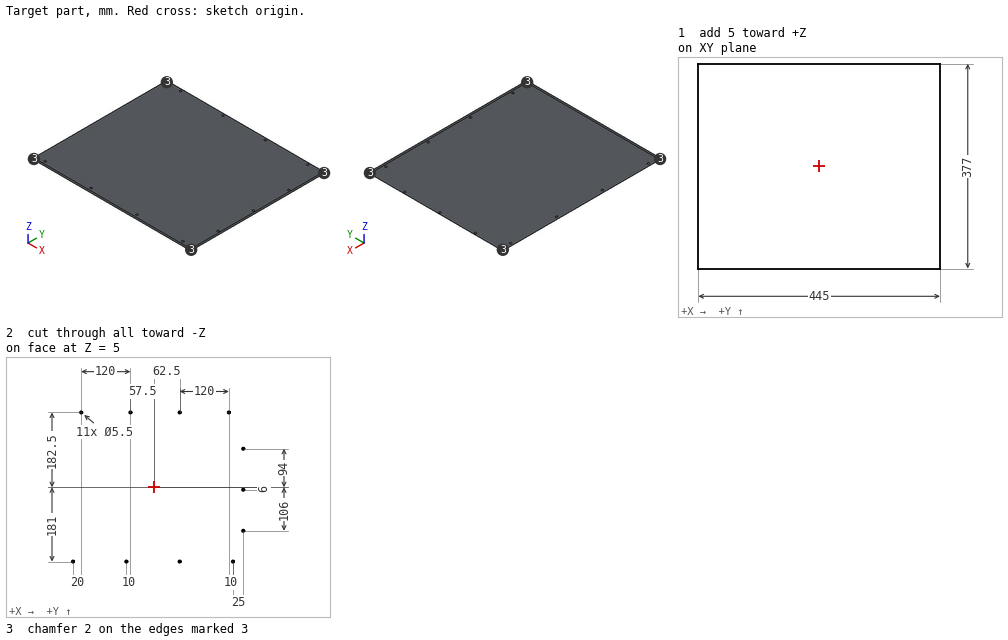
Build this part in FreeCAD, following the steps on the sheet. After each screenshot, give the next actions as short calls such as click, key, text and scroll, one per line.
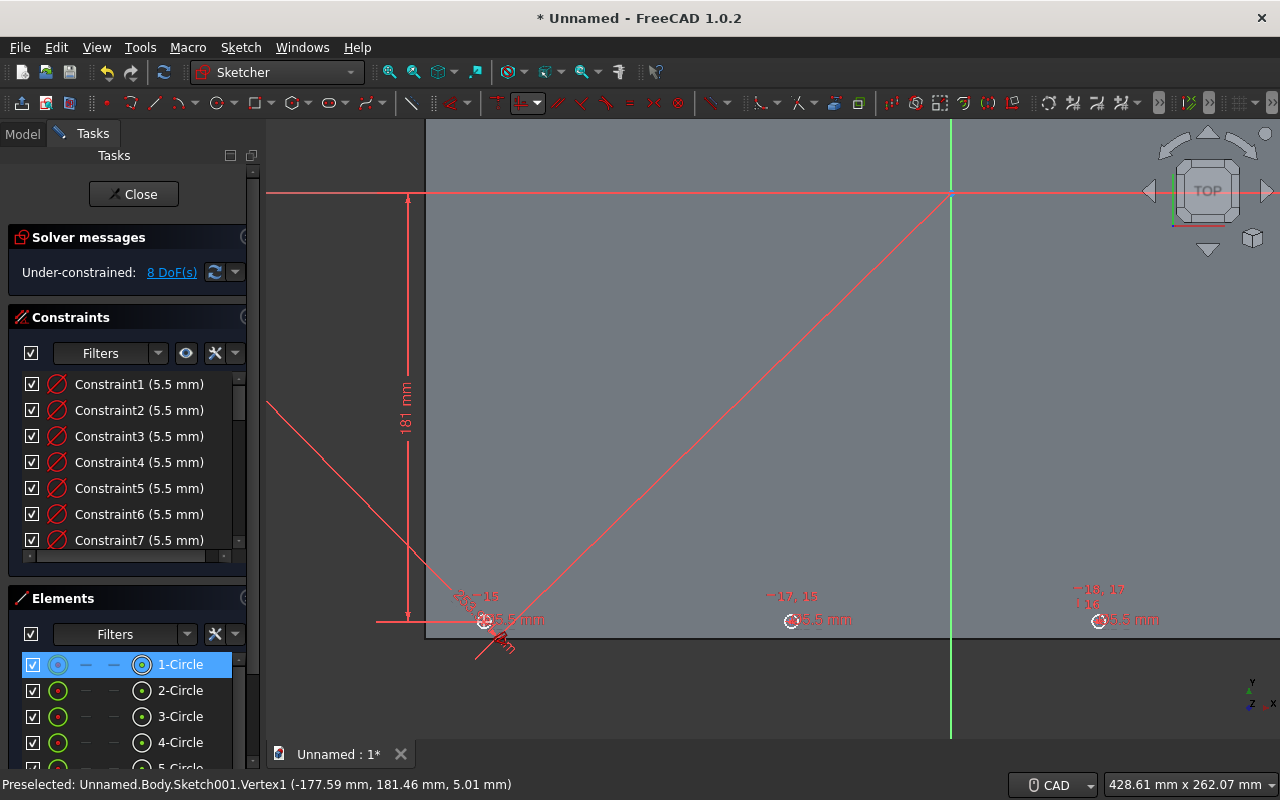
click(484, 622)
click(508, 656)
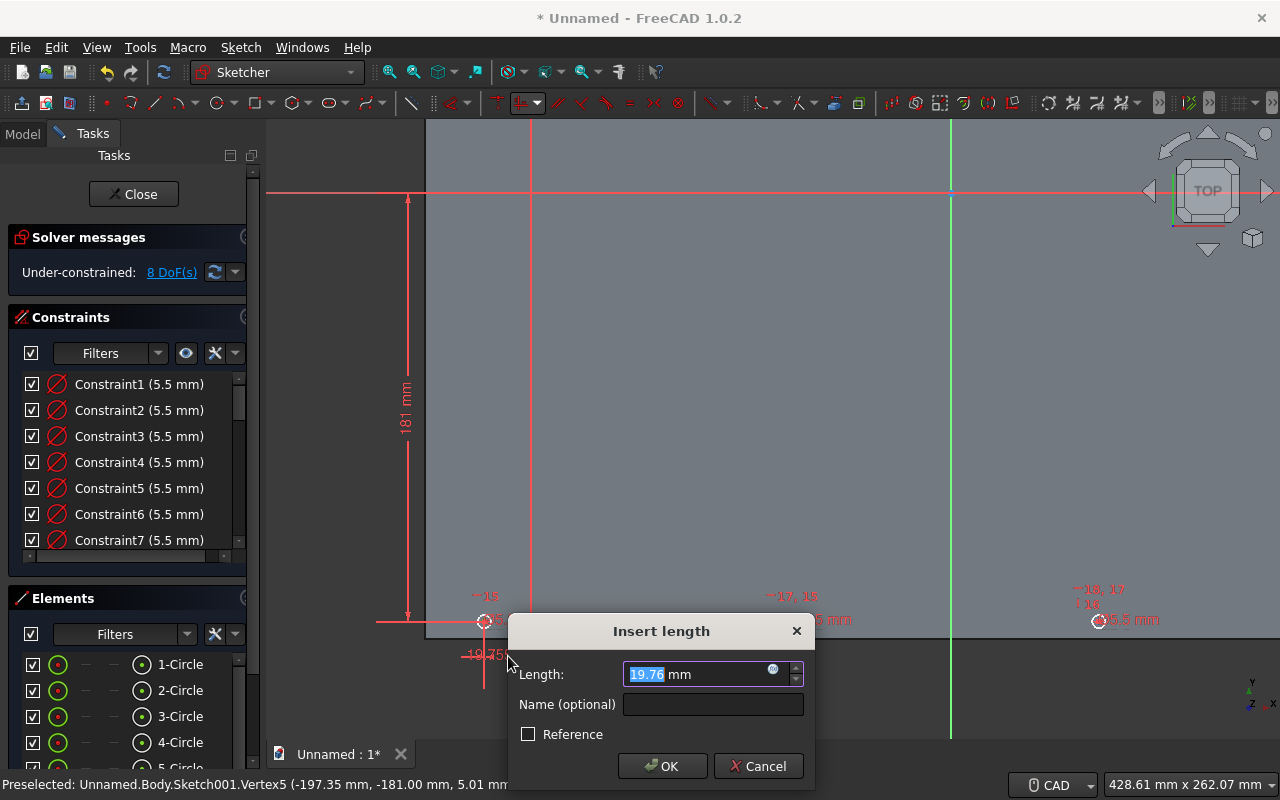
text(20)
key(Return)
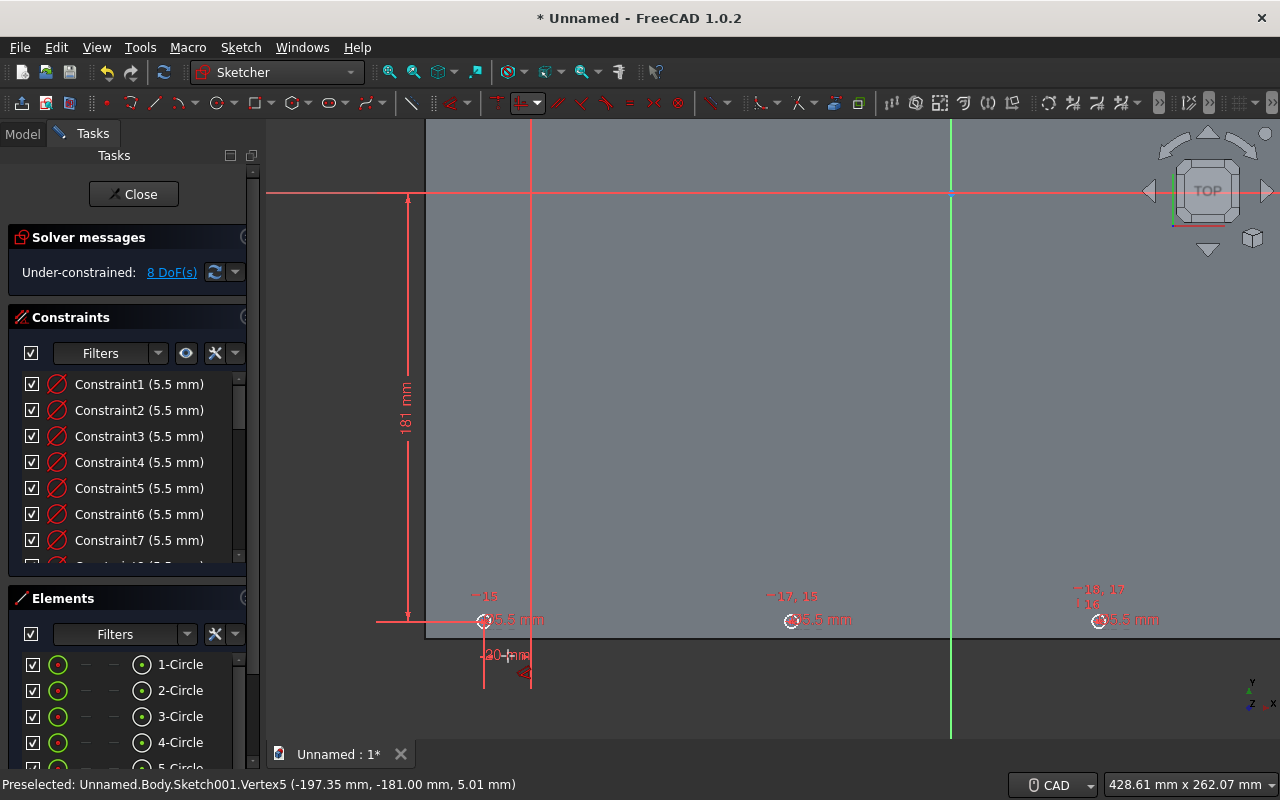
scroll(484, 623, down, 4)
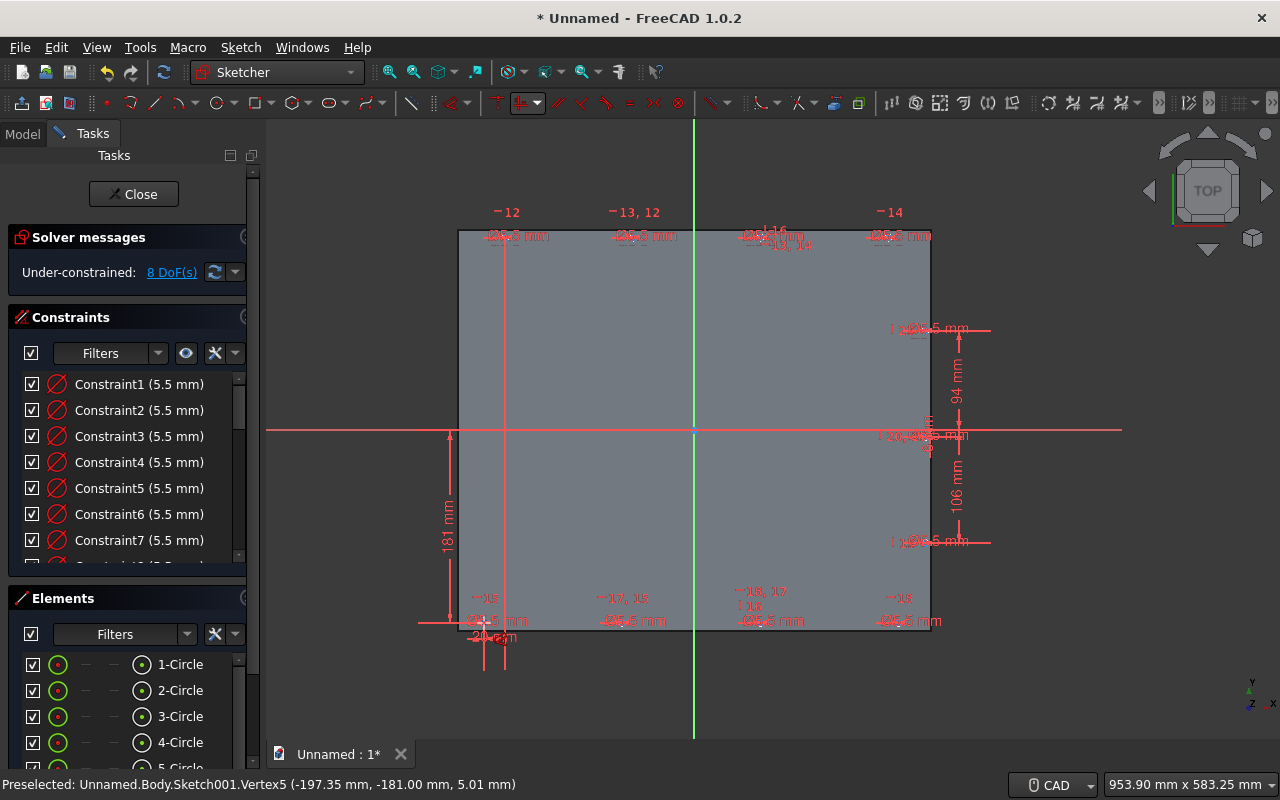
scroll(633, 238, up, 7)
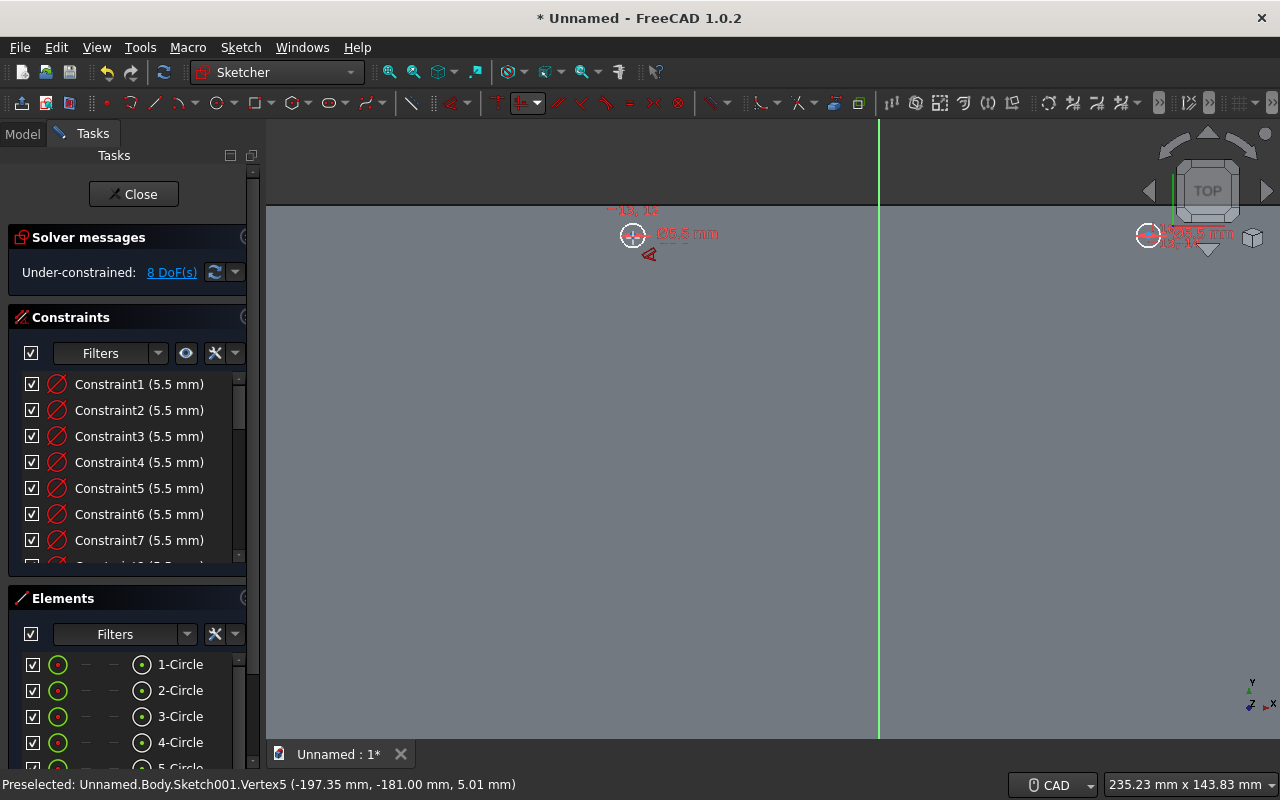
click(633, 236)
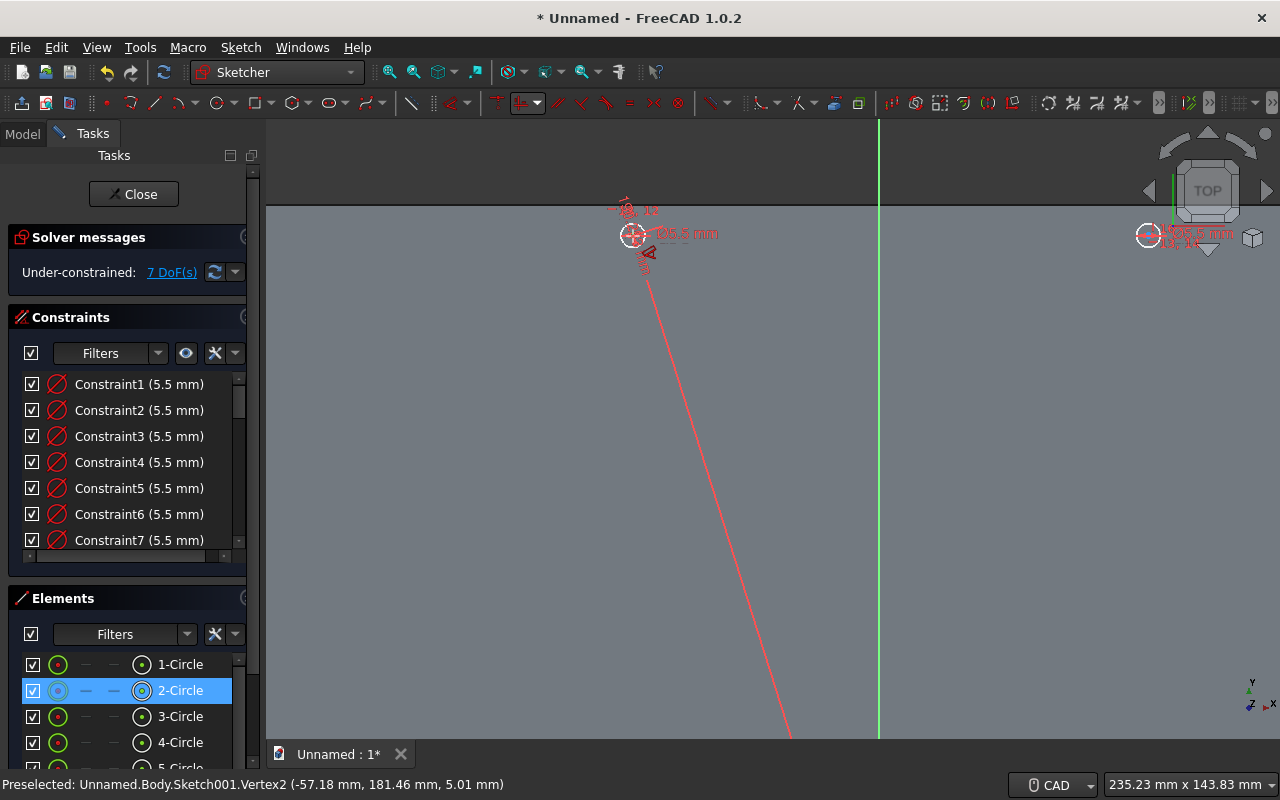
scroll(633, 237, down, 7)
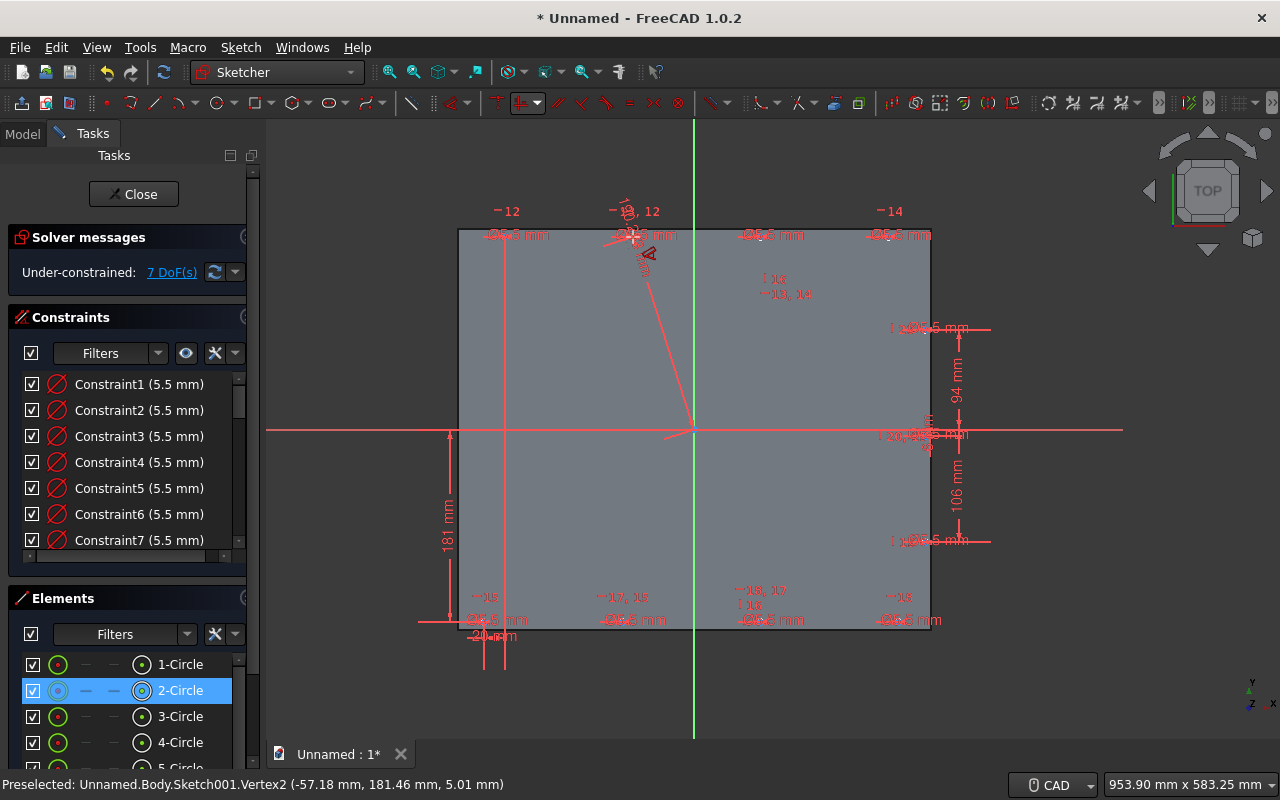
scroll(622, 622, up, 7)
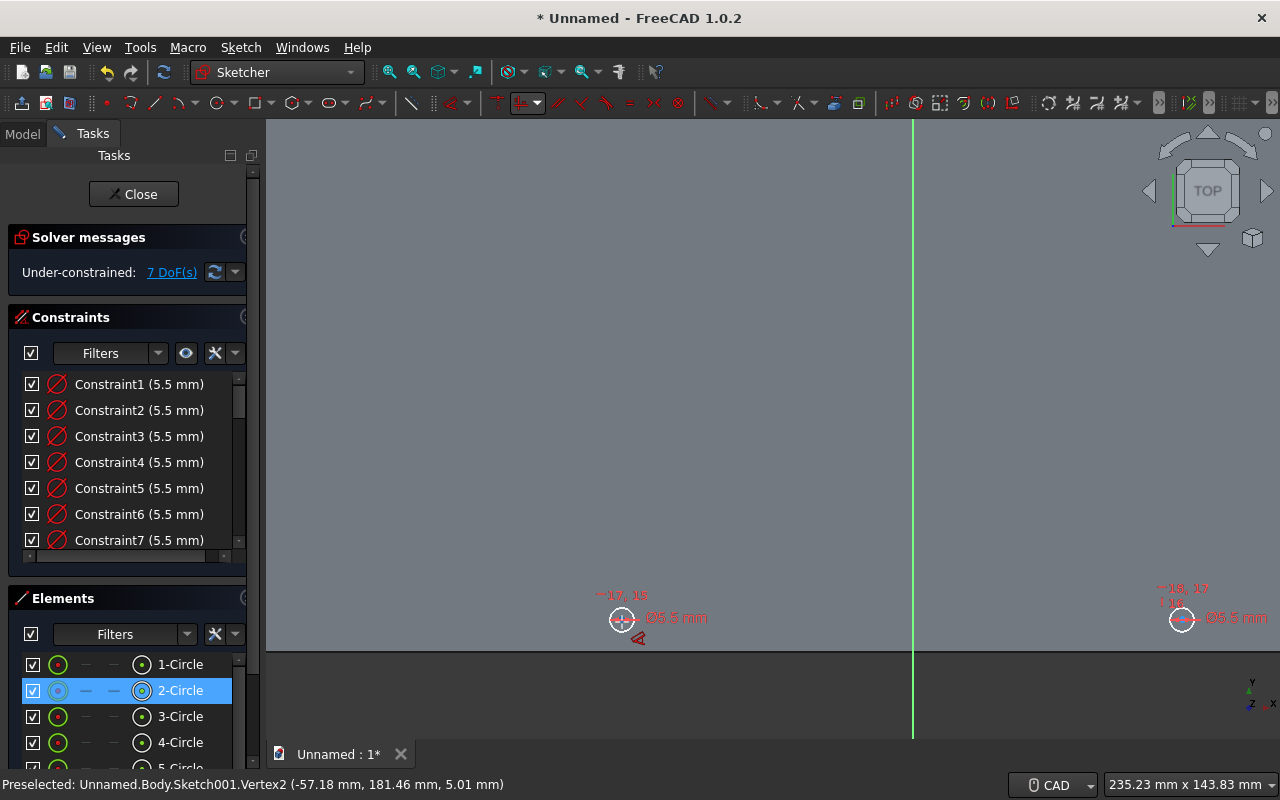
click(622, 620)
click(644, 654)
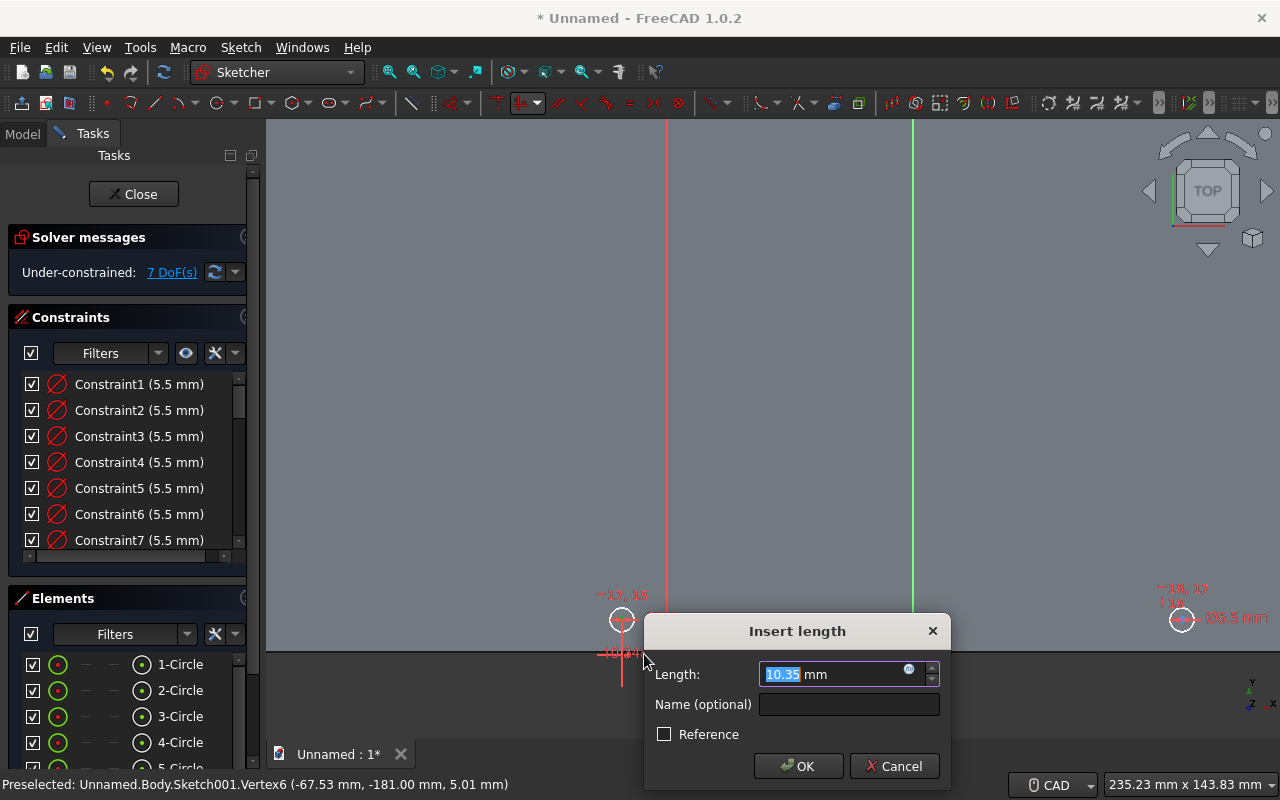
text(10)
key(Return)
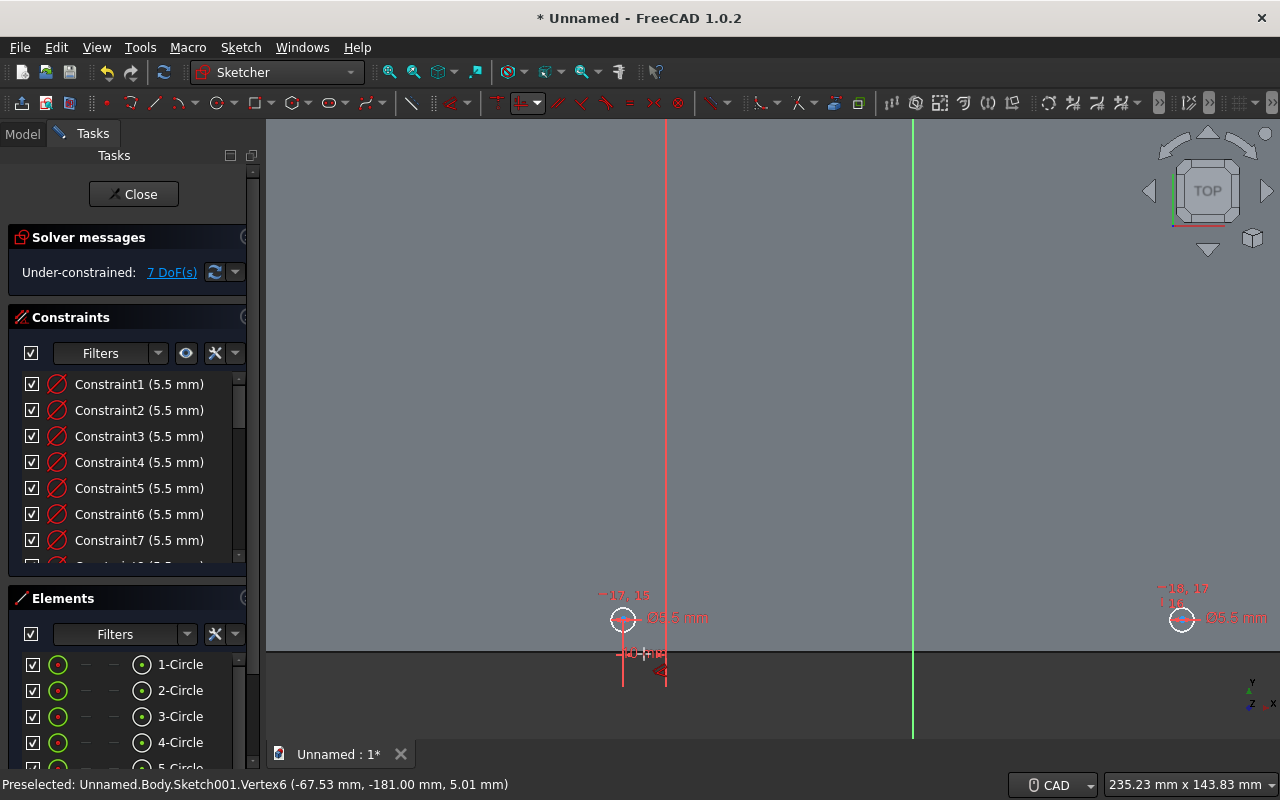
scroll(622, 623, down, 7)